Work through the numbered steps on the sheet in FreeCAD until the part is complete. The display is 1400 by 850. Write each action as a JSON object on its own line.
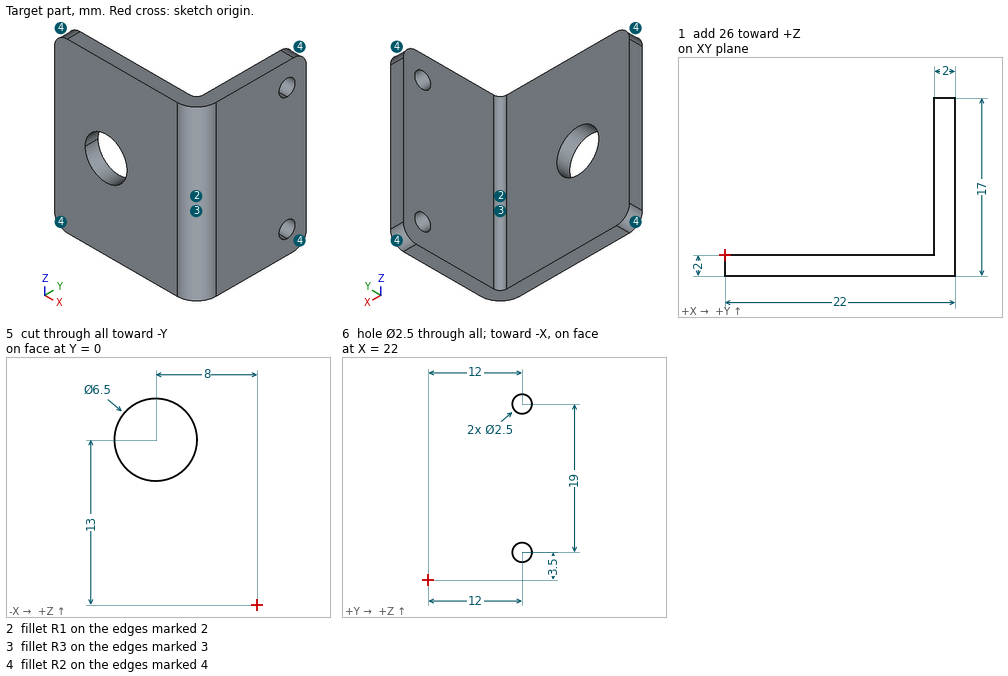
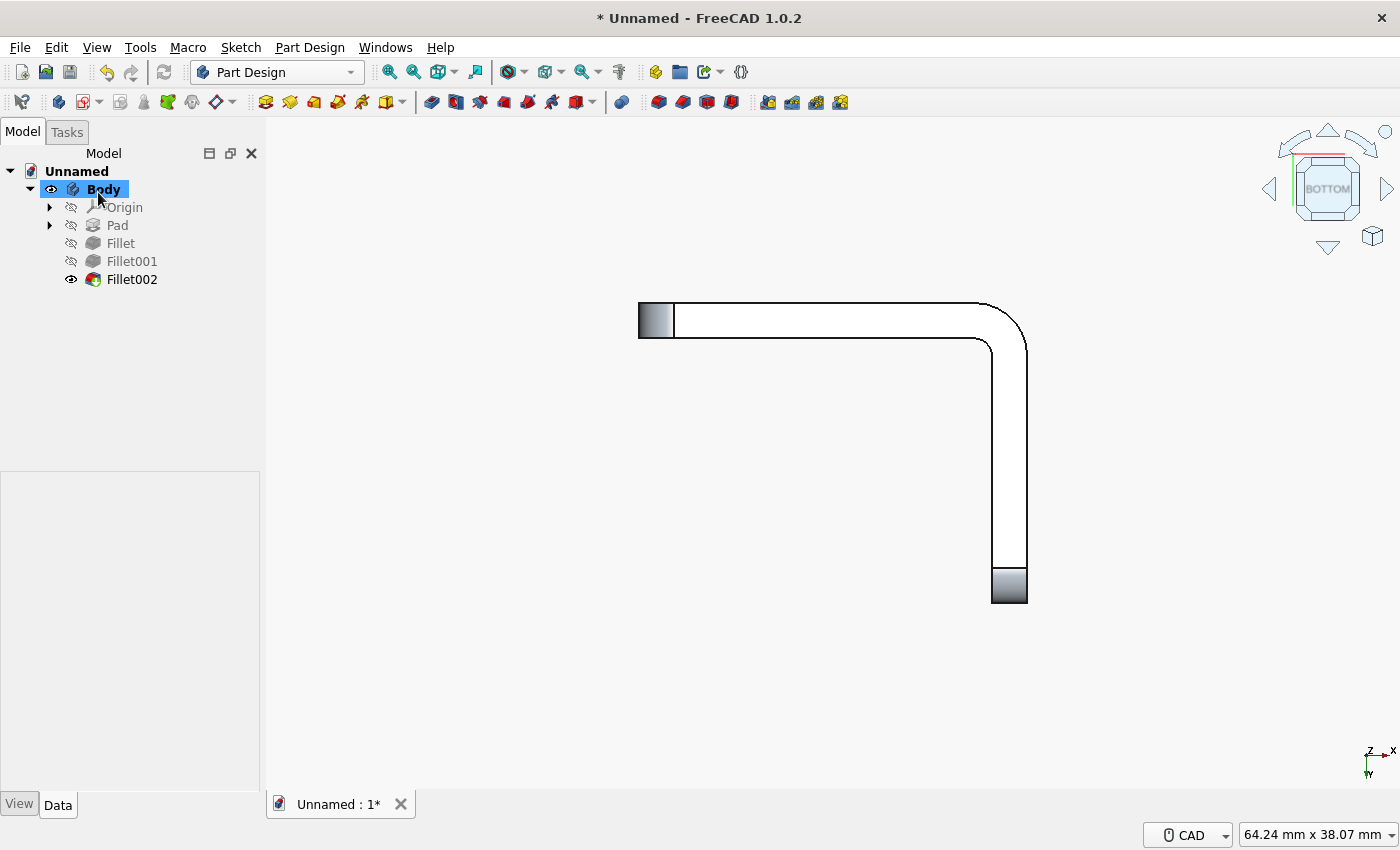
{"action": "key", "text": "4"}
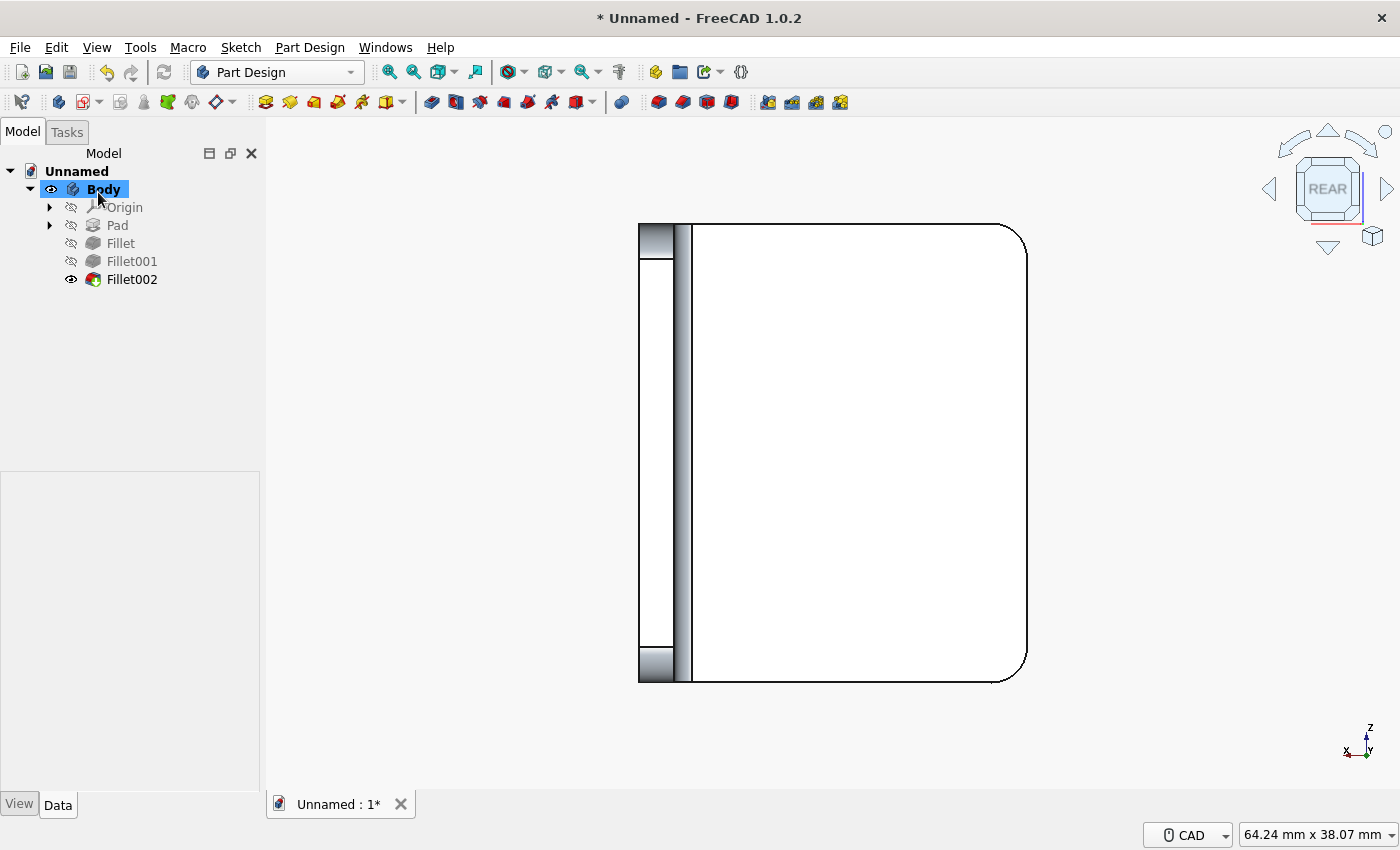
{"action": "left_click", "coordinate": [859, 452]}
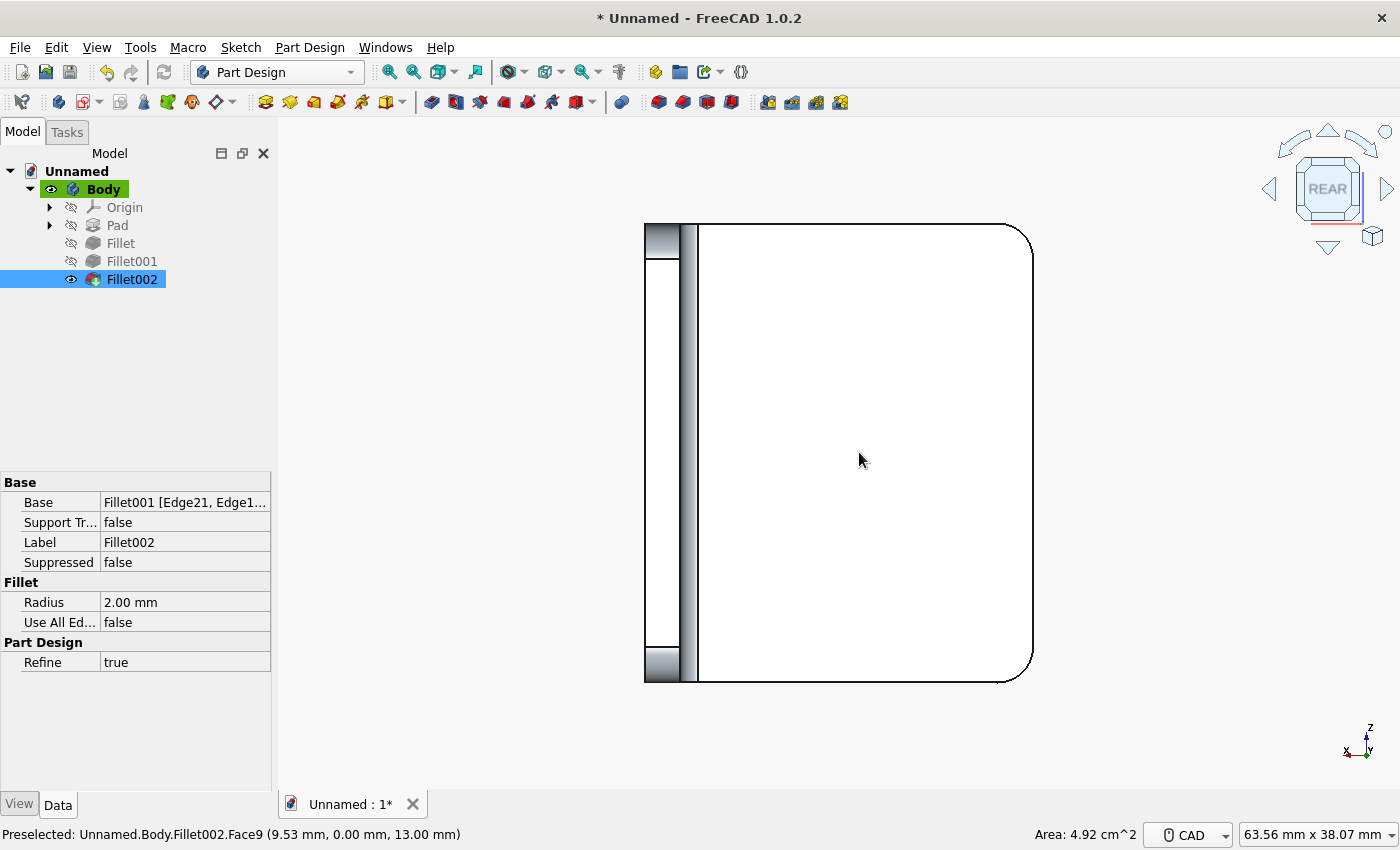
{"action": "left_click", "coordinate": [84, 102]}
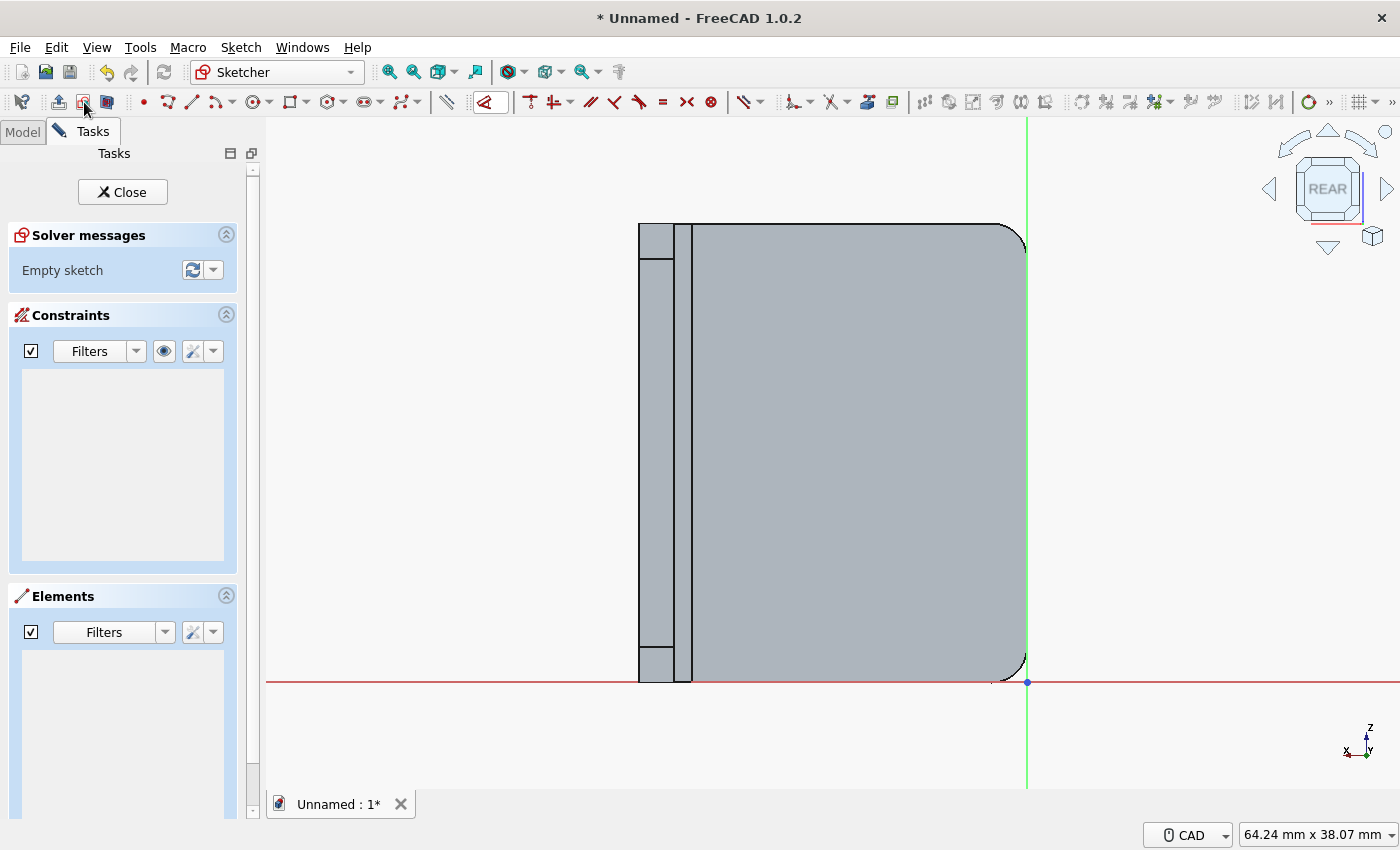
{"action": "scroll", "coordinate": [926, 453], "scroll_direction": "up", "scroll_amount": 7}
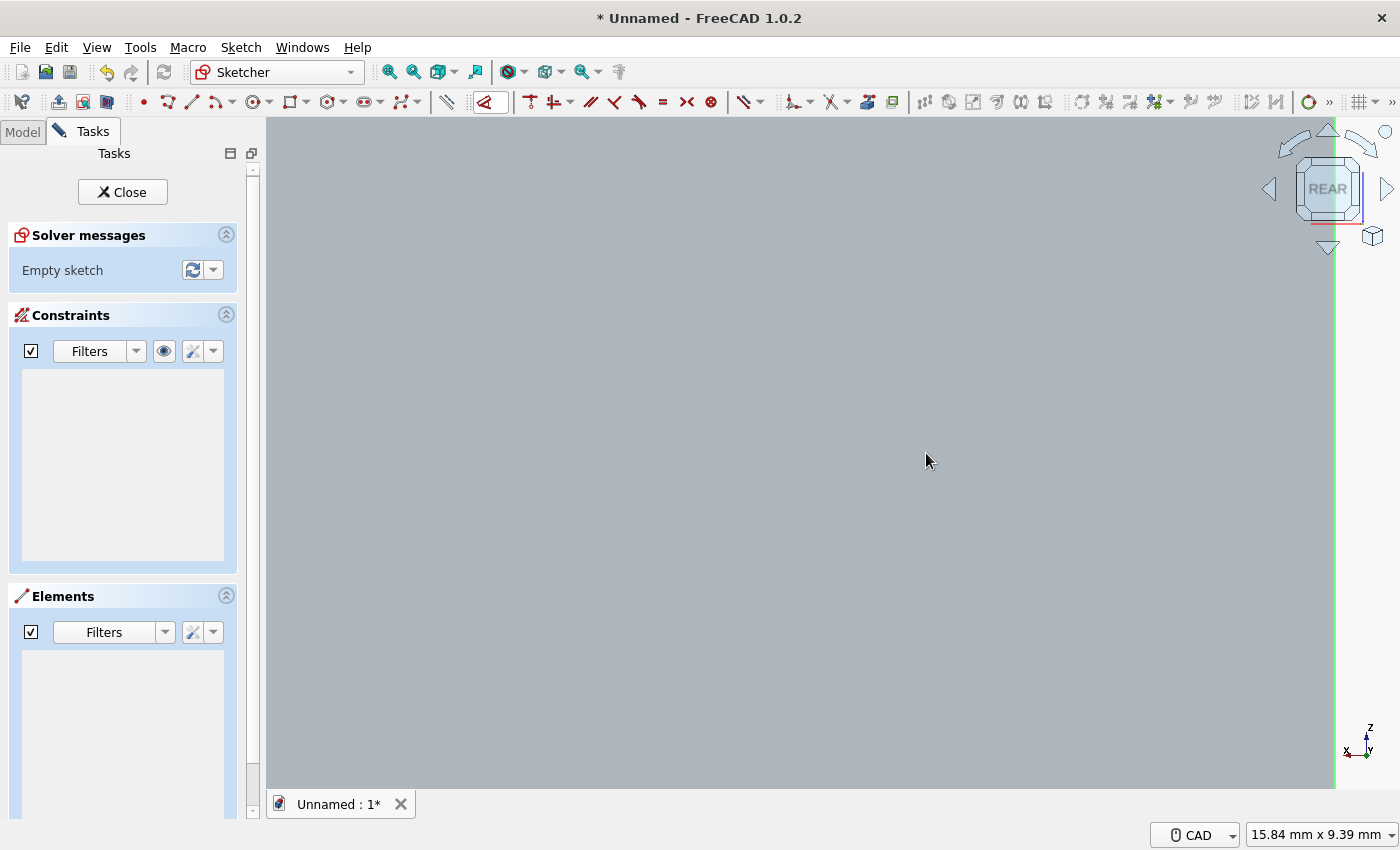
{"action": "key", "text": "g c"}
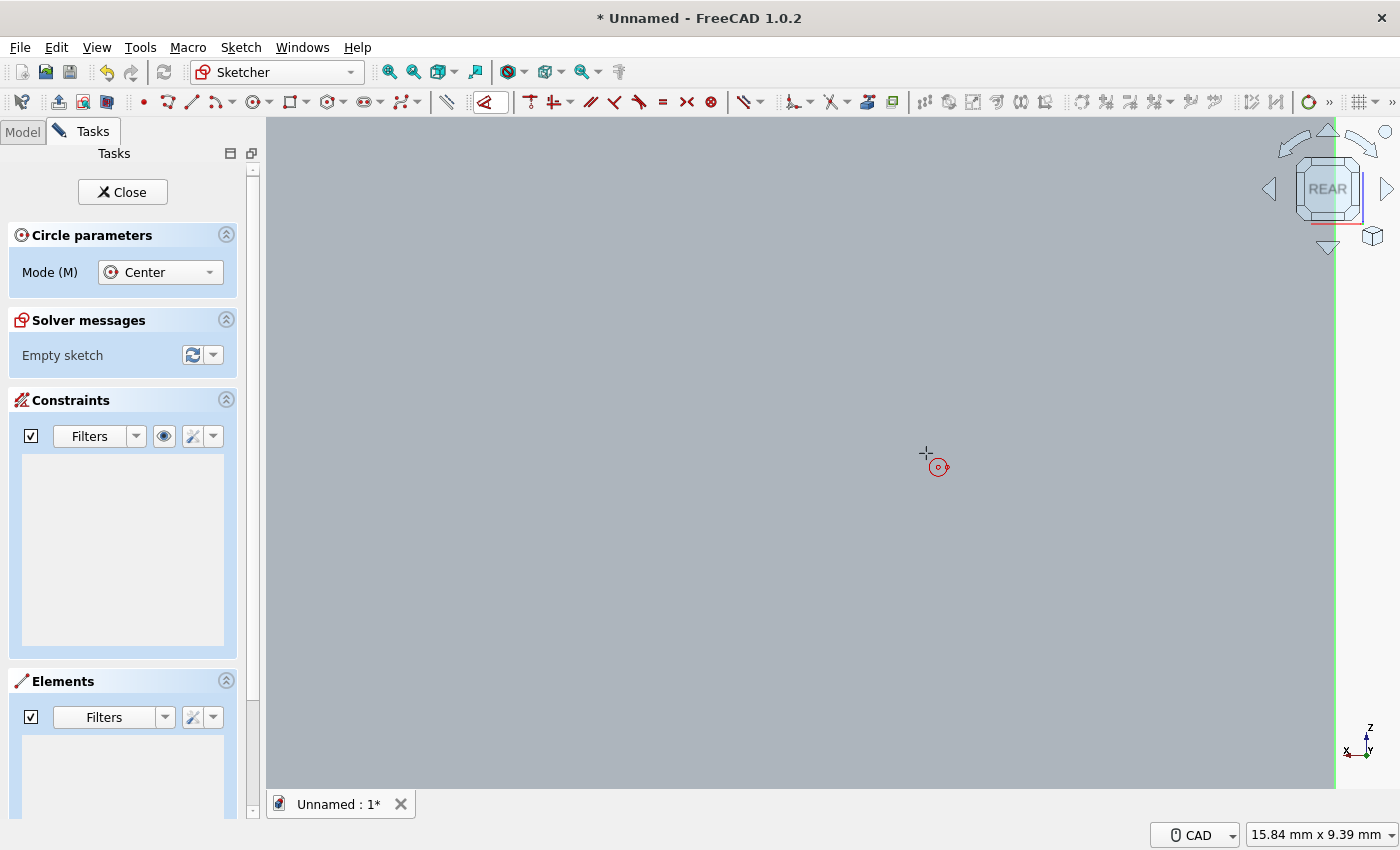
{"action": "left_click", "coordinate": [762, 451]}
{"action": "mouse_move", "coordinate": [926, 287]}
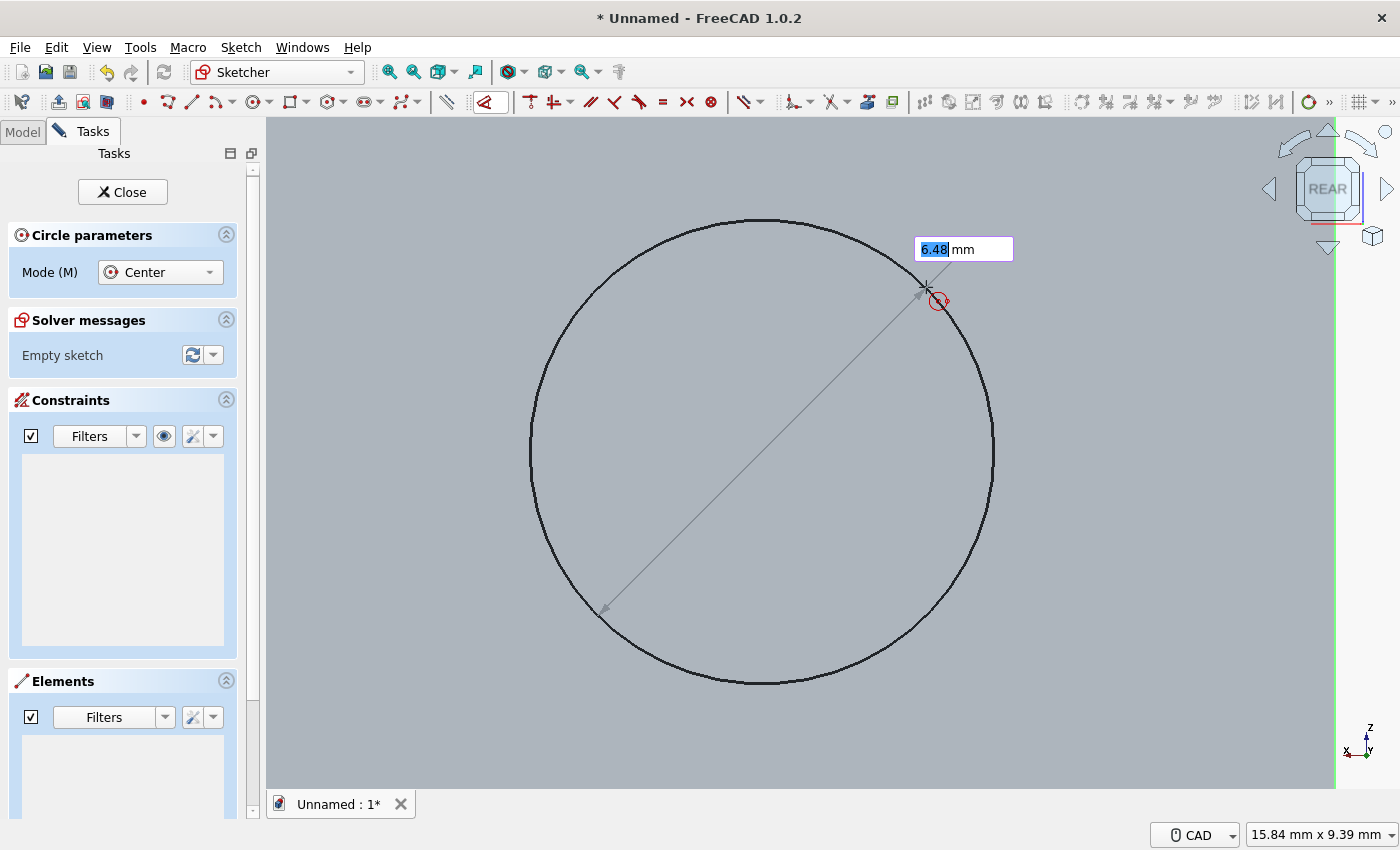
{"action": "type", "text": "6.5"}
{"action": "key", "text": "Return"}
{"action": "key", "text": "Escape"}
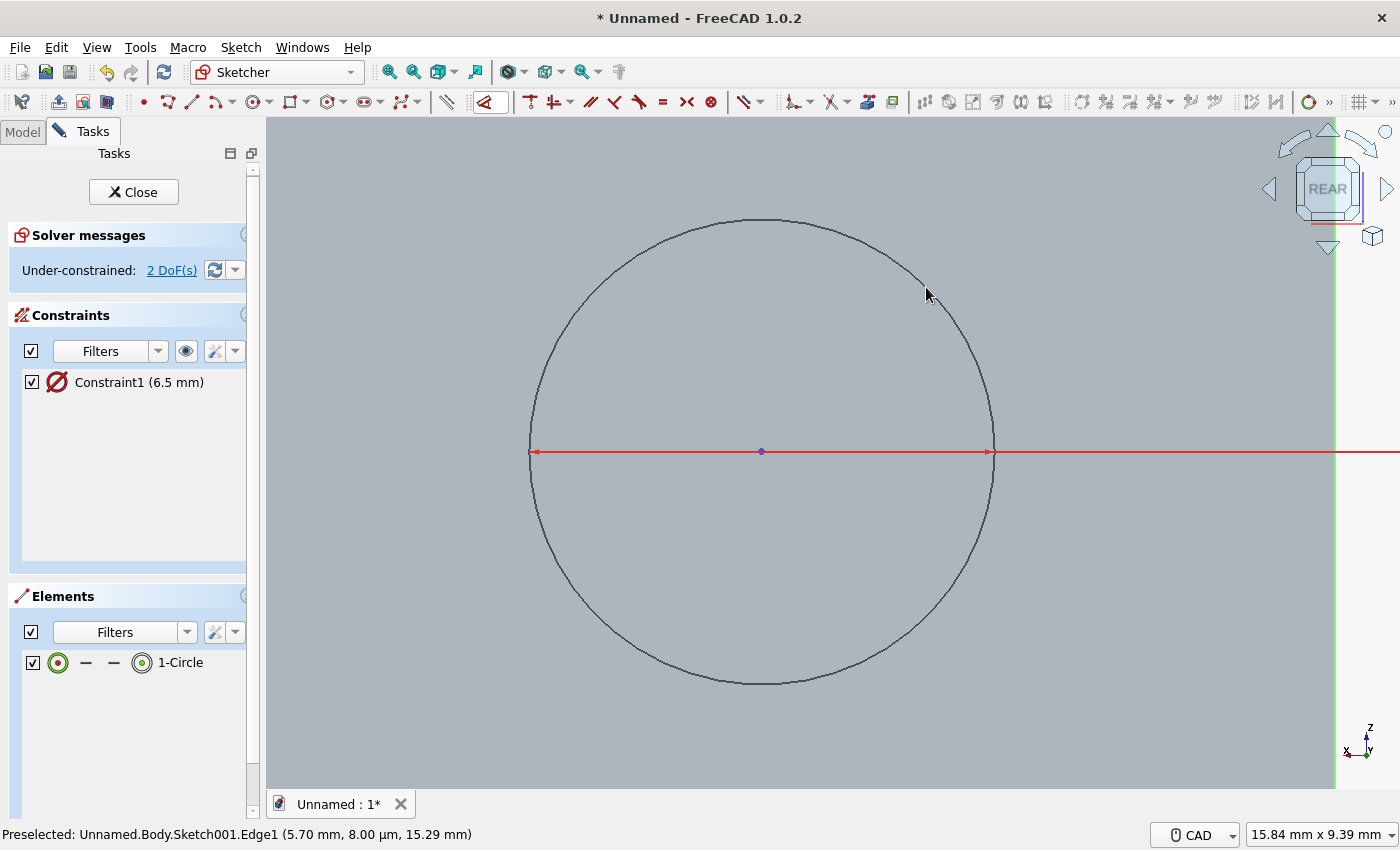
{"action": "key", "text": "d"}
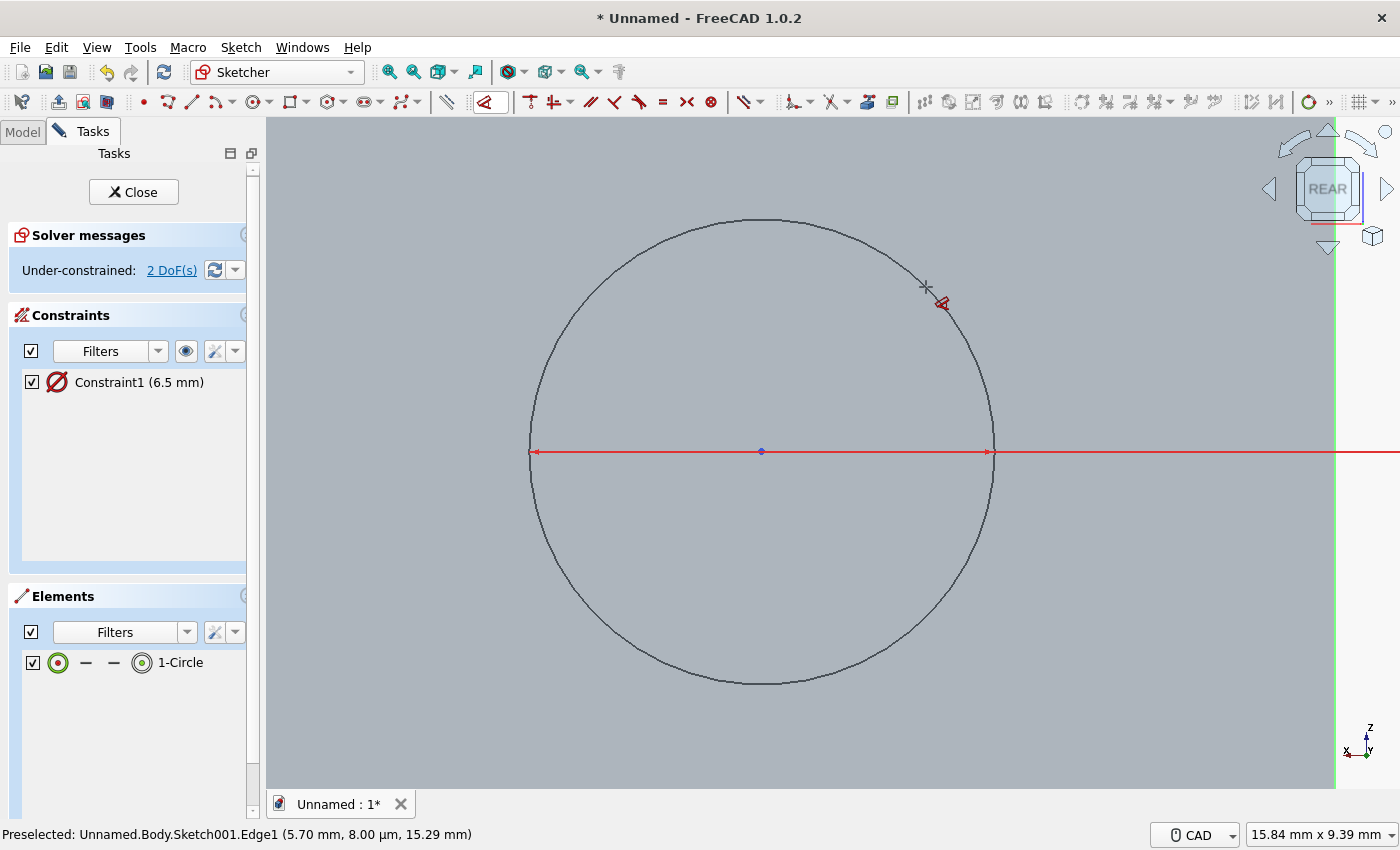
{"action": "left_click", "coordinate": [762, 452]}
{"action": "left_click", "coordinate": [890, 418]}